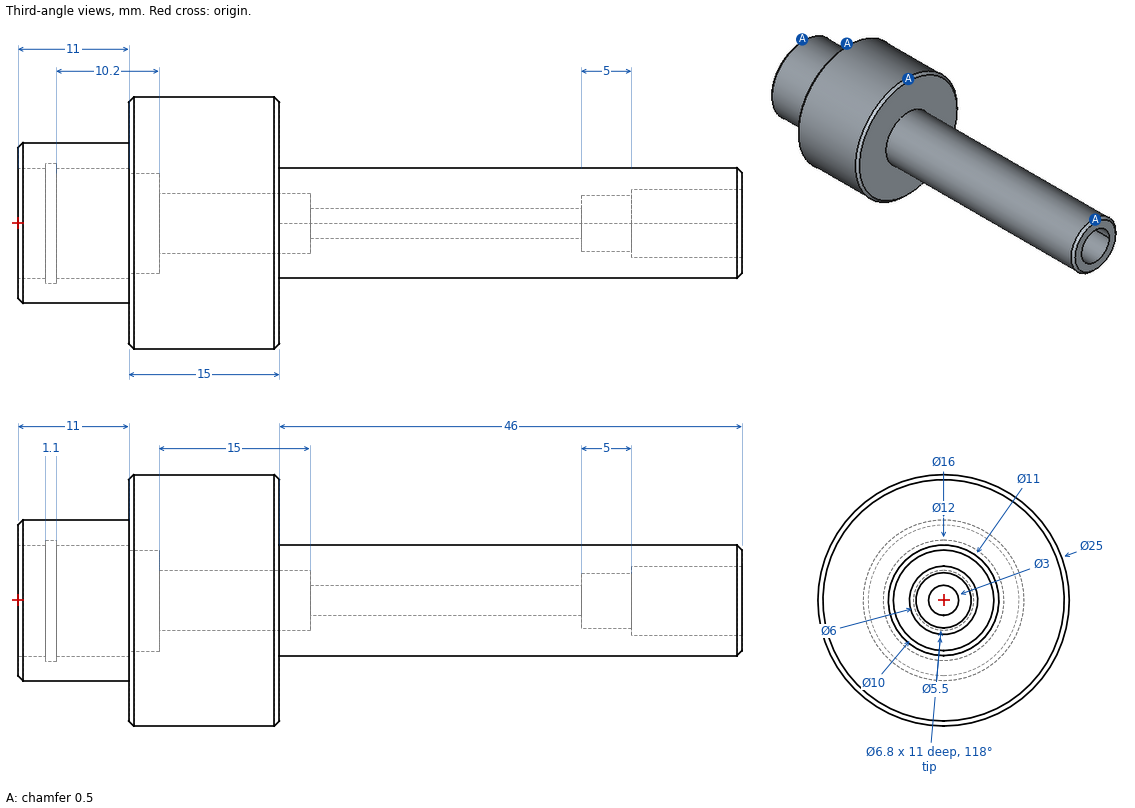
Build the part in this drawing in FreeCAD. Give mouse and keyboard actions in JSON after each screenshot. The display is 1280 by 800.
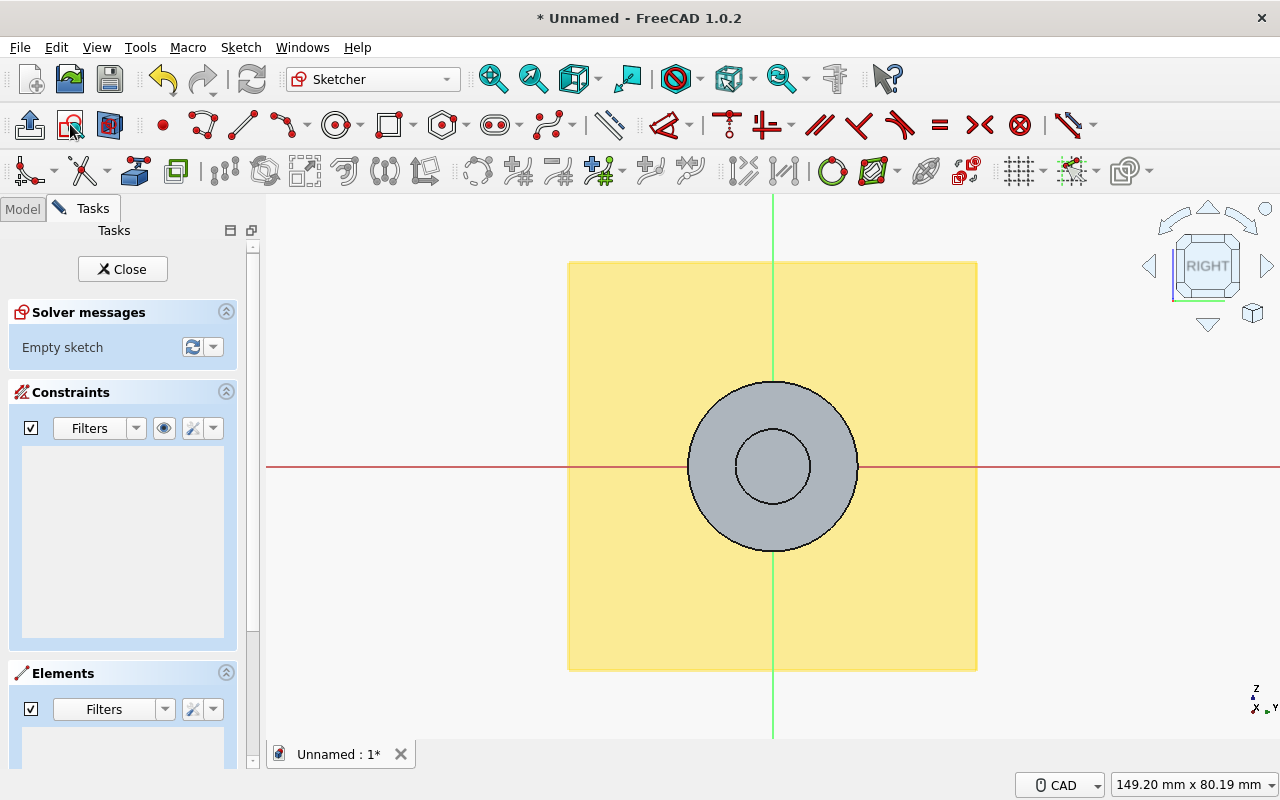
{"action": "key", "text": "q s"}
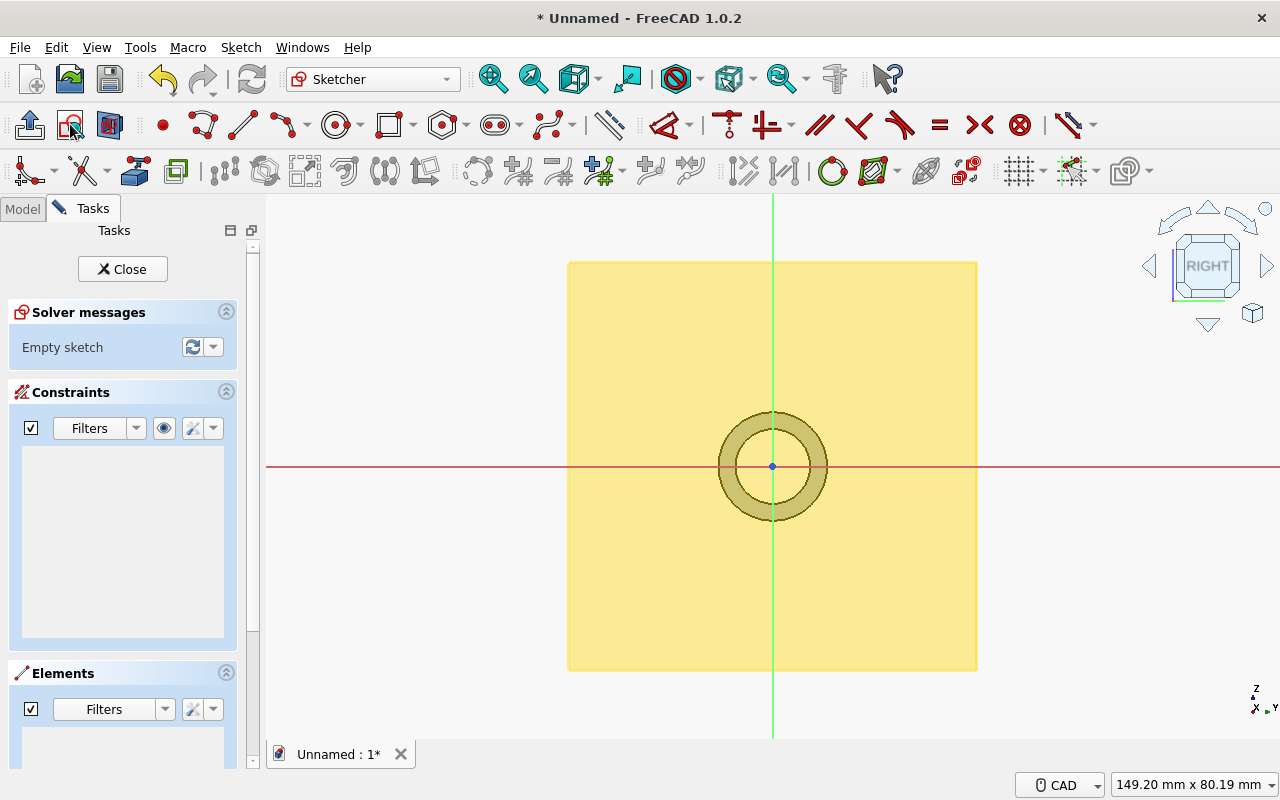
{"action": "scroll", "coordinate": [795, 466], "scroll_direction": "up", "scroll_amount": 7}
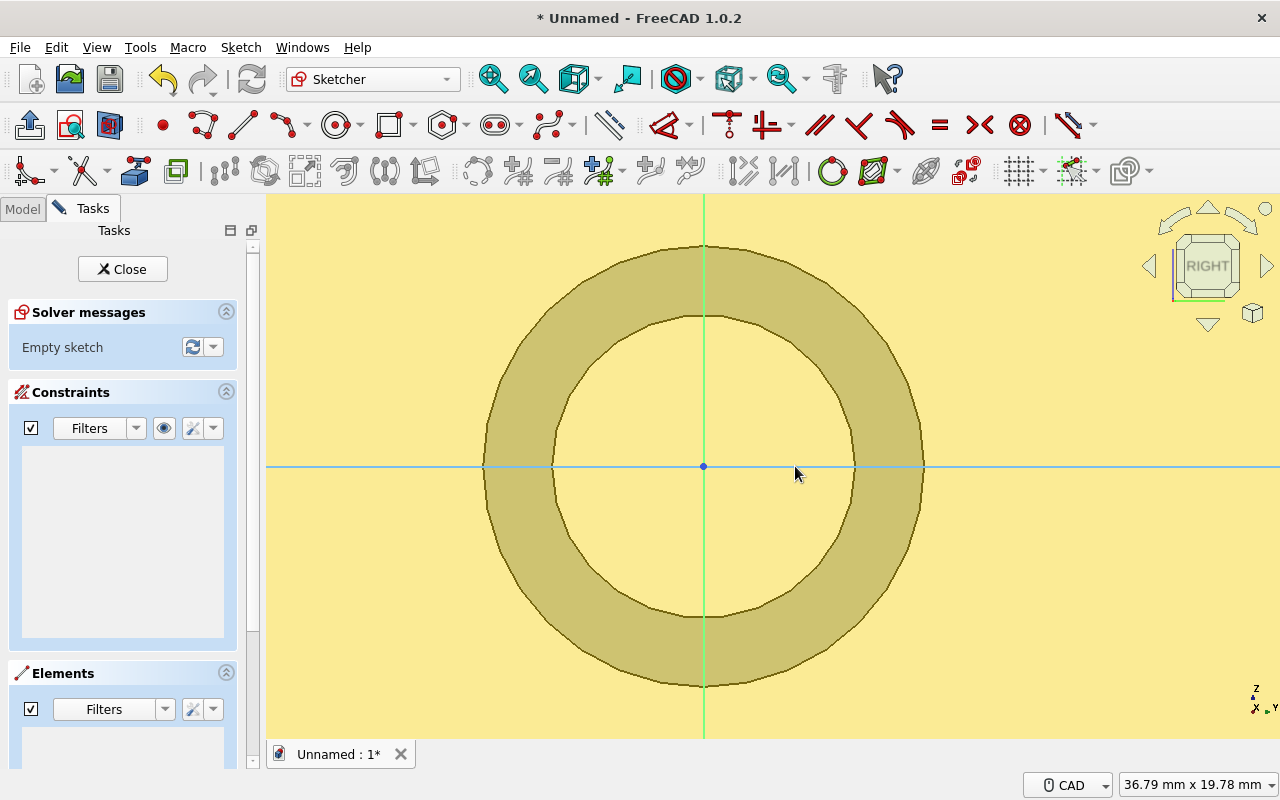
{"action": "left_click", "coordinate": [336, 126]}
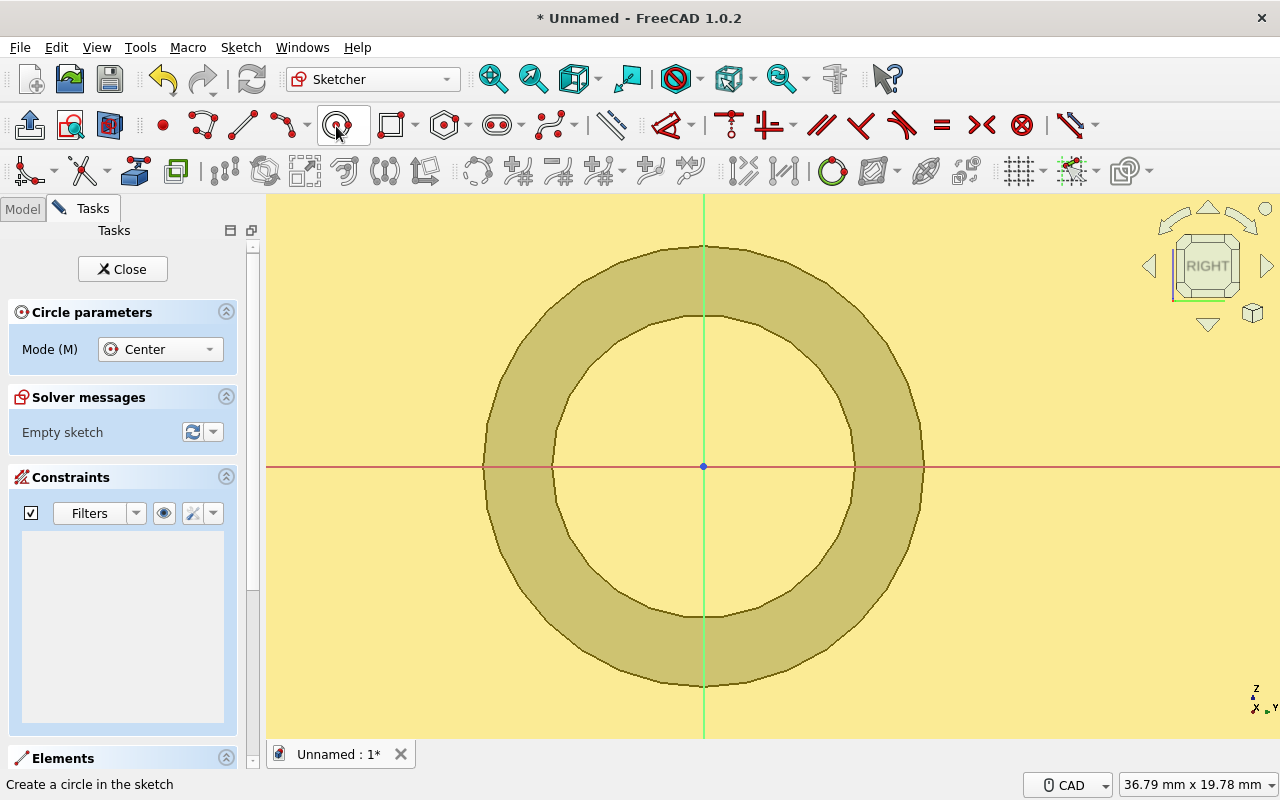
{"action": "left_click", "coordinate": [704, 466]}
{"action": "mouse_move", "coordinate": [821, 350]}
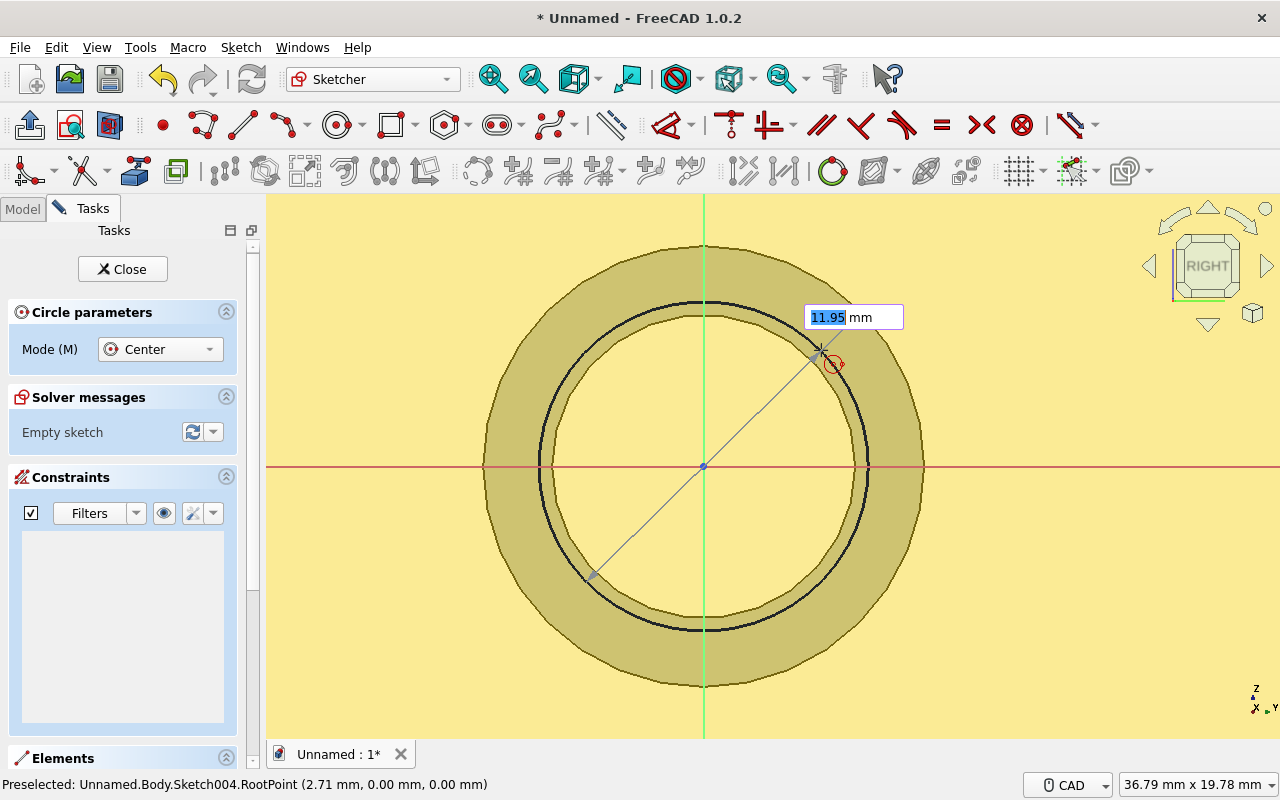
{"action": "type", "text": "12"}
{"action": "key", "text": "Return"}
{"action": "key", "text": "Escape"}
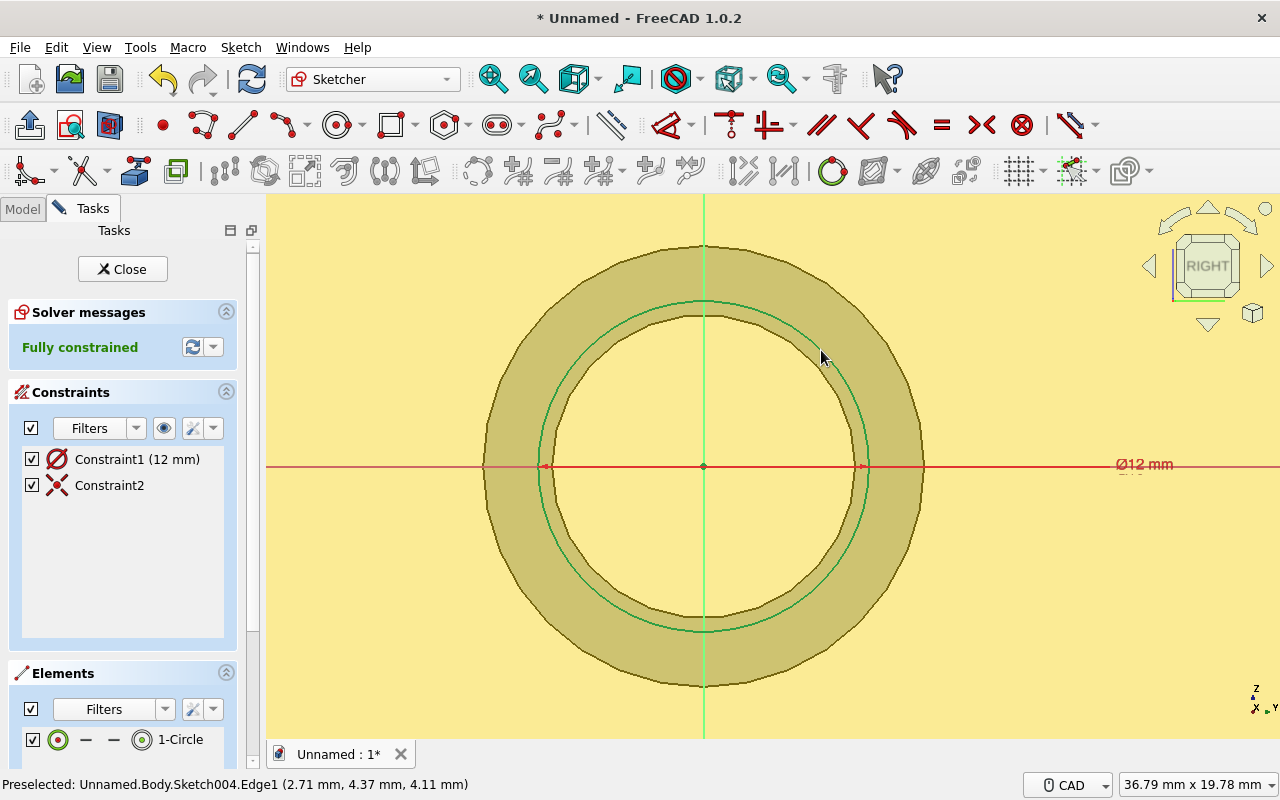
{"action": "left_click", "coordinate": [123, 269]}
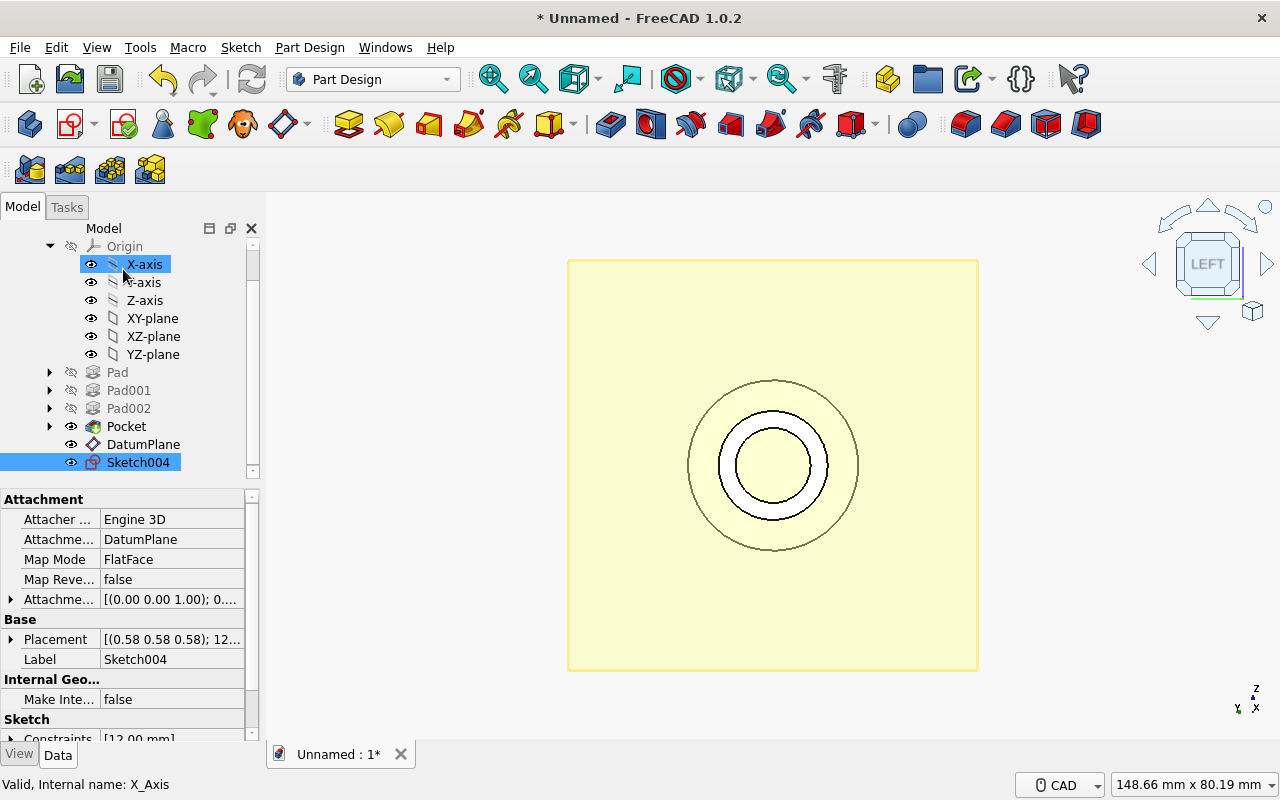
{"action": "left_click", "coordinate": [612, 124]}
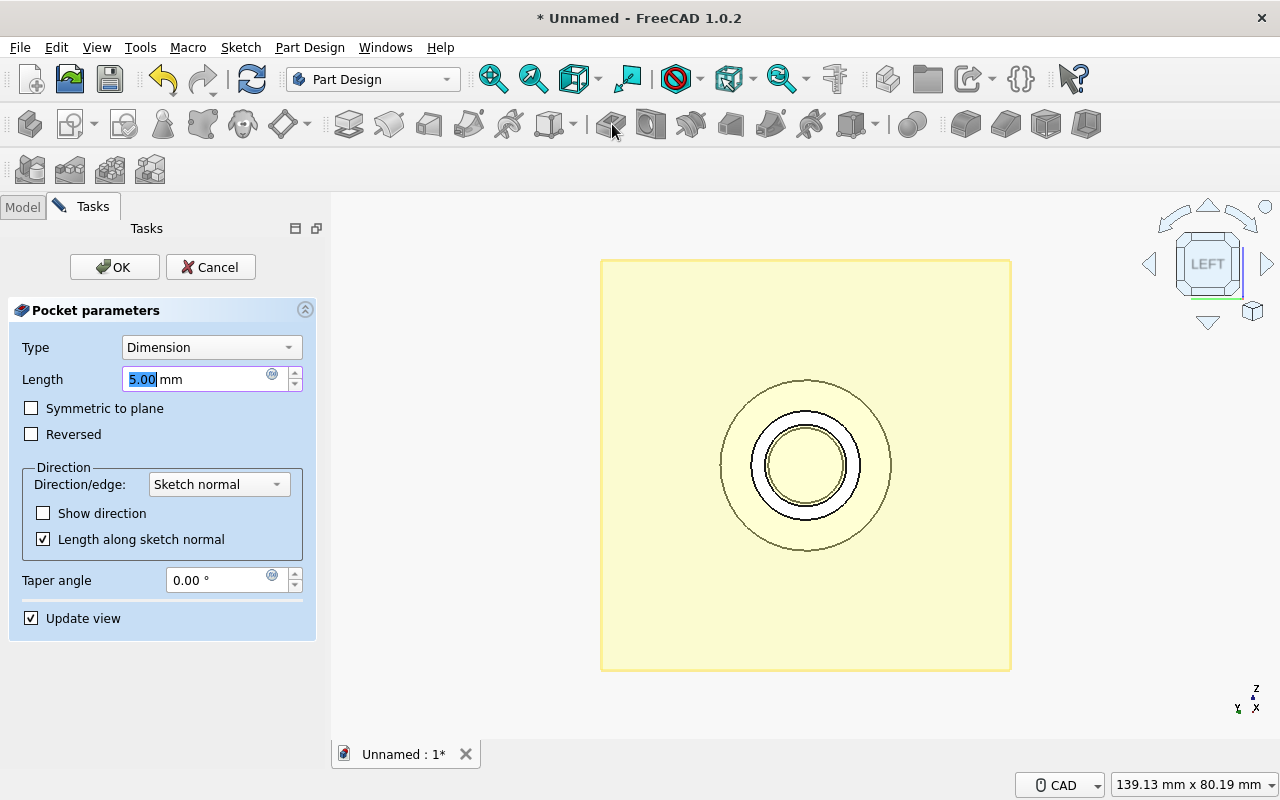
{"action": "type", "text": "1.1"}
{"action": "key", "text": "Tab"}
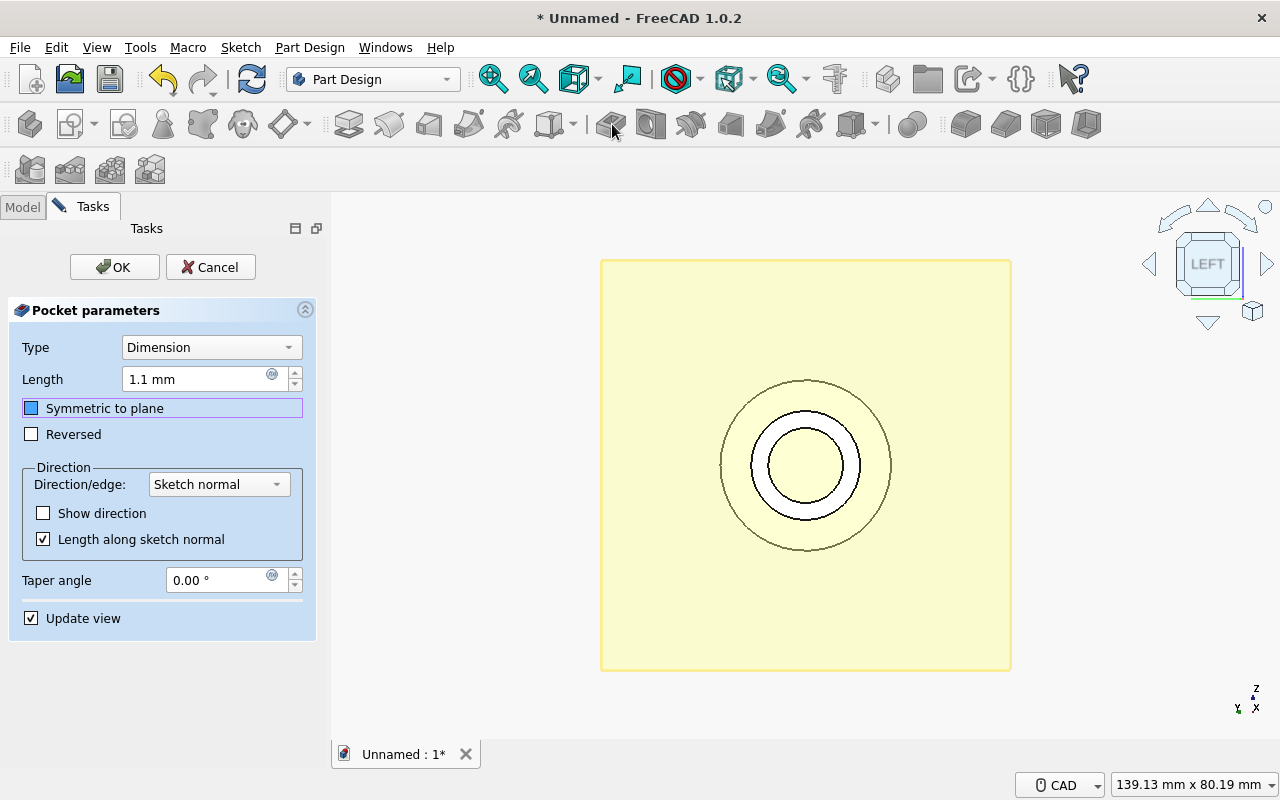
{"action": "left_click", "coordinate": [30, 434]}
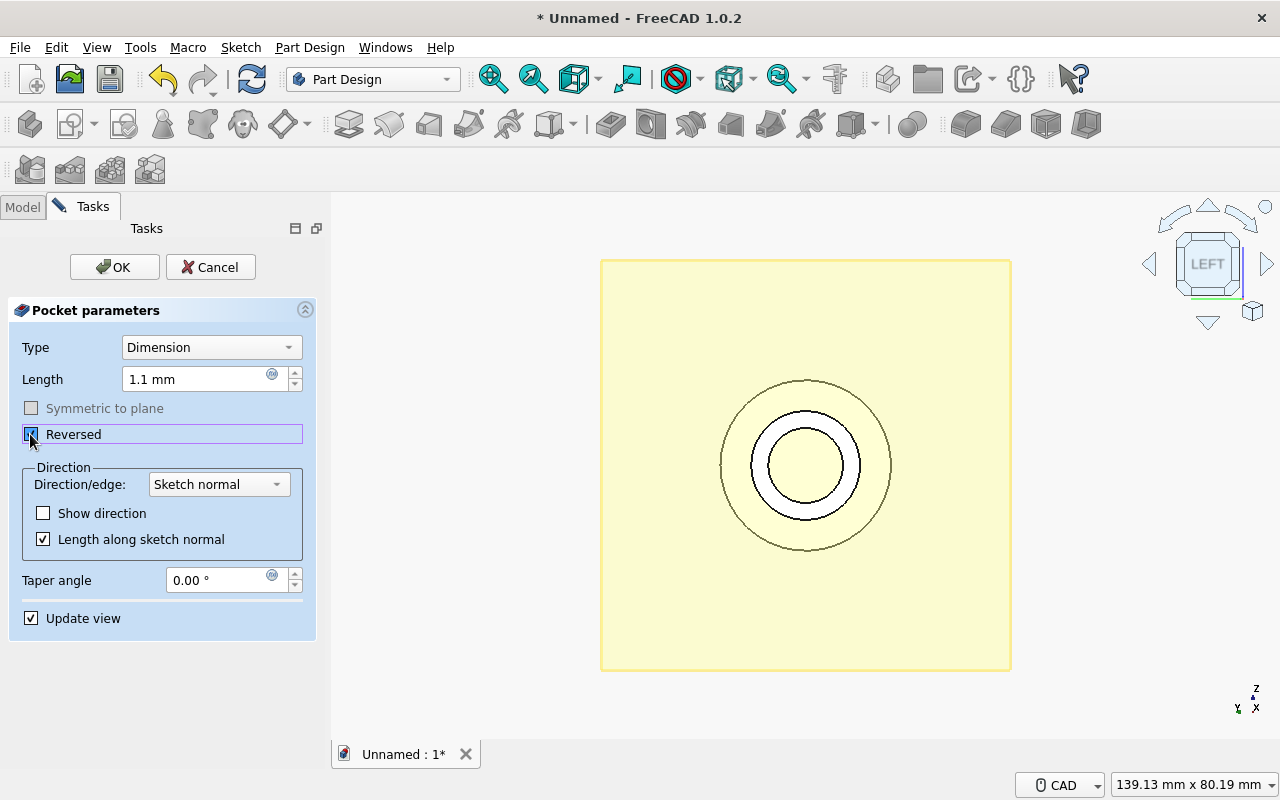
{"action": "left_click", "coordinate": [115, 267]}